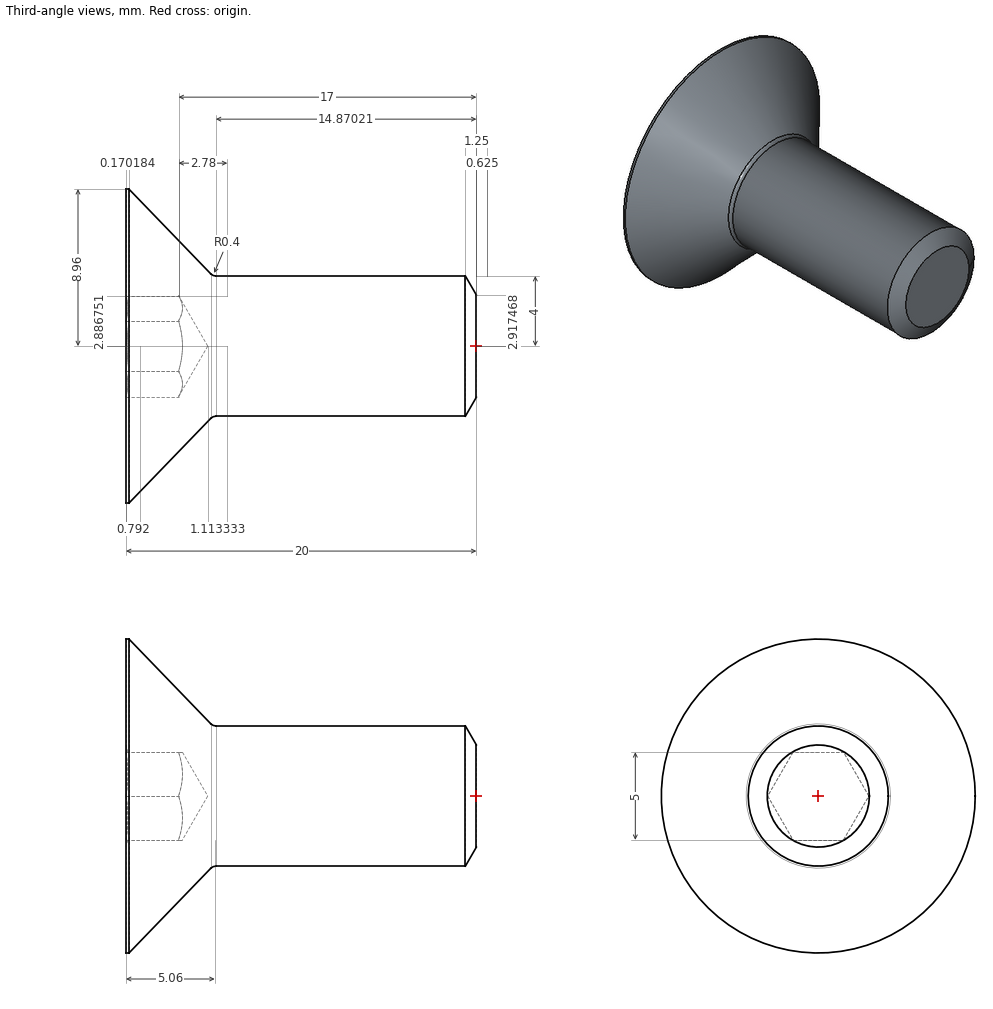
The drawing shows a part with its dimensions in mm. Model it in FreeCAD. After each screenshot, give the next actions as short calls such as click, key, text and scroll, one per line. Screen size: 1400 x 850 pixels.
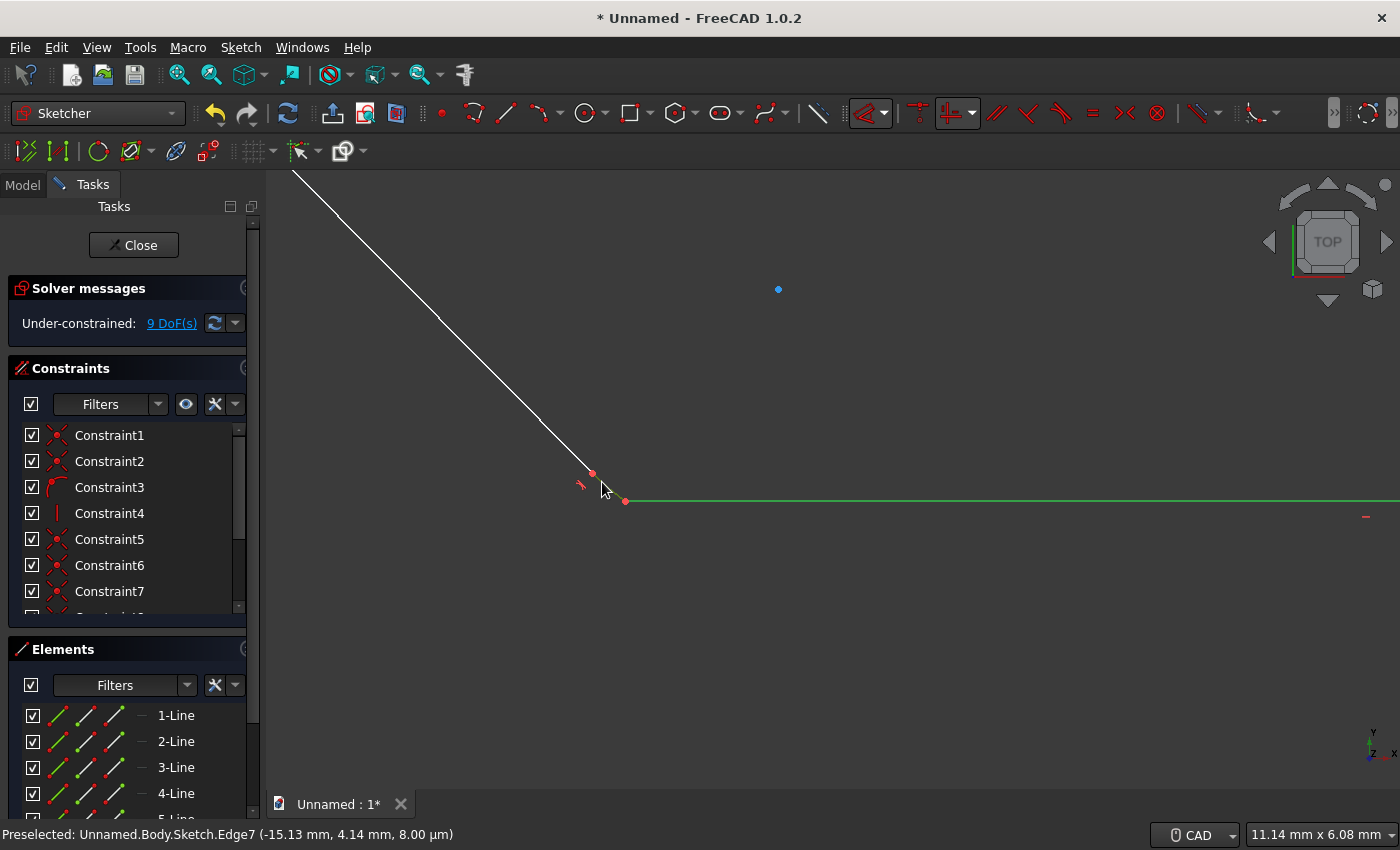
click(1062, 114)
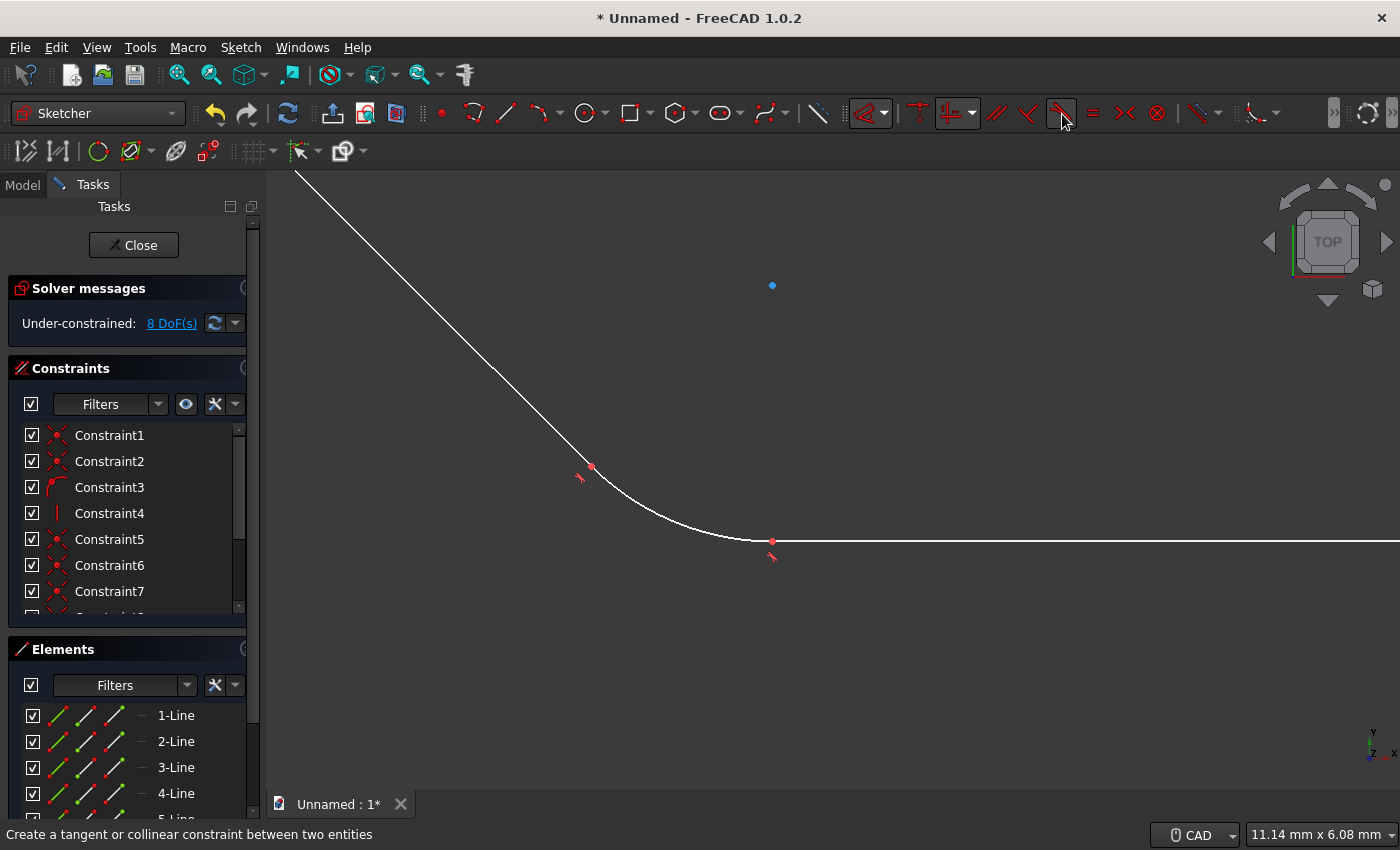
scroll(611, 494, down, 6)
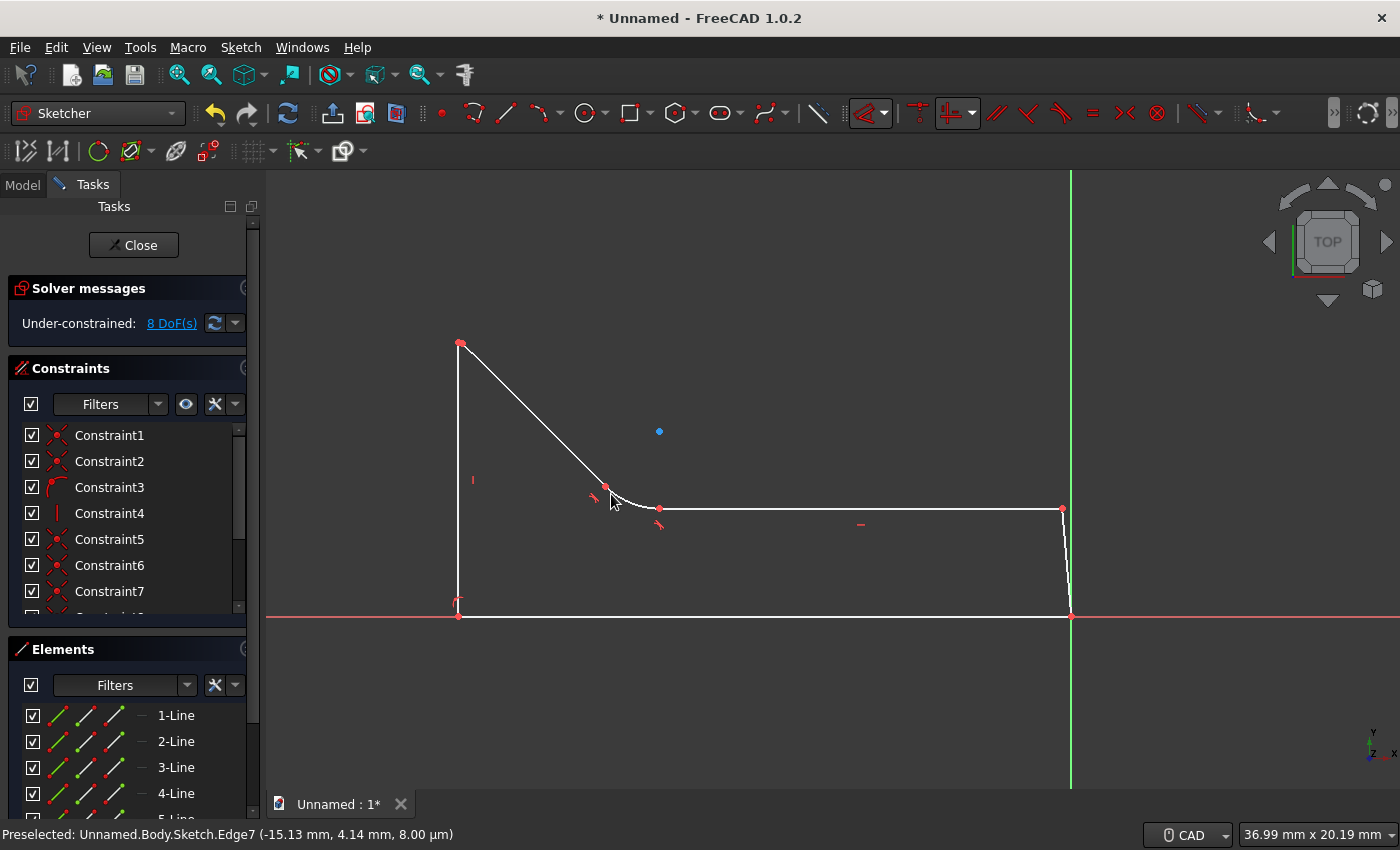
scroll(460, 343, up, 10)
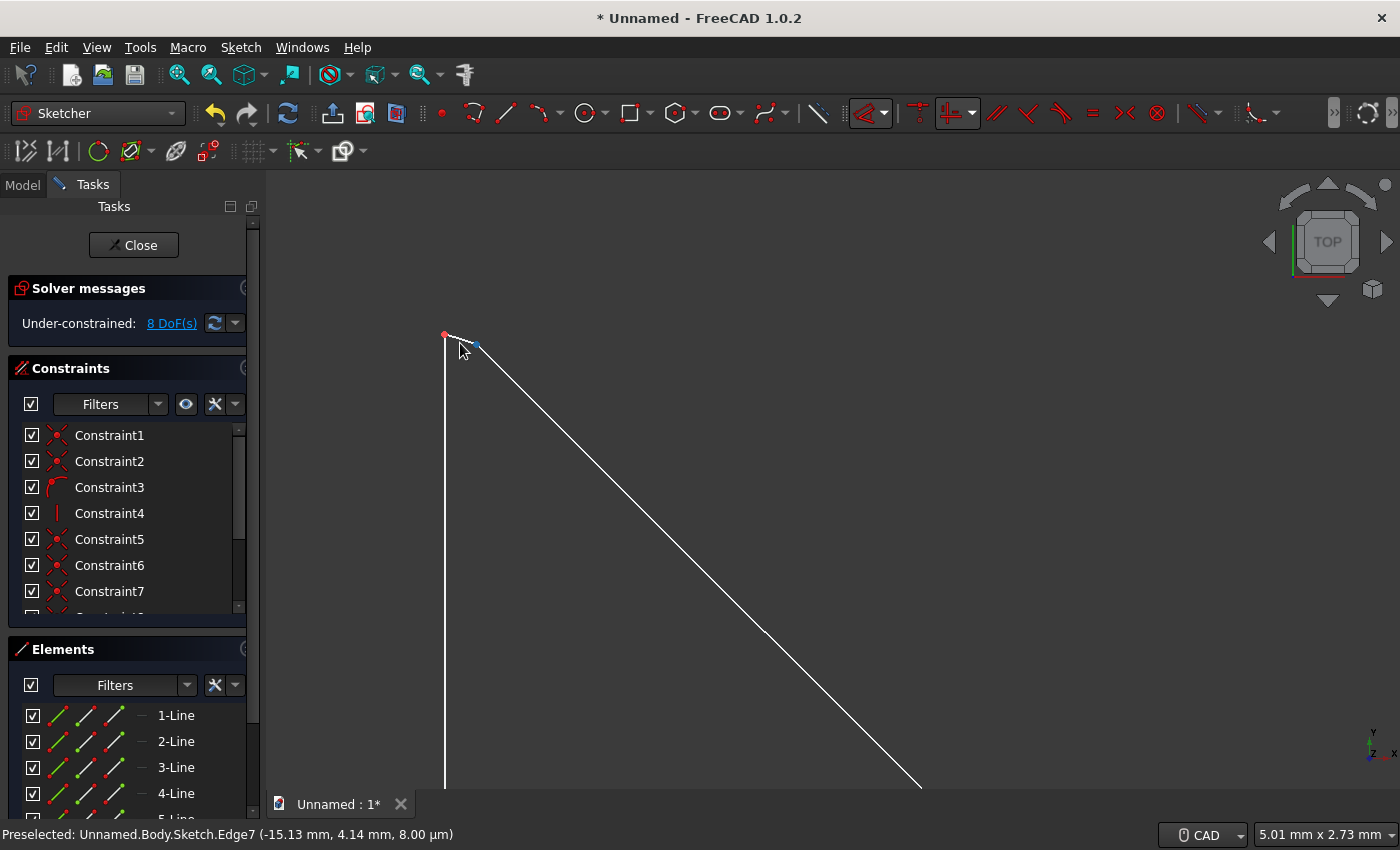
click(460, 339)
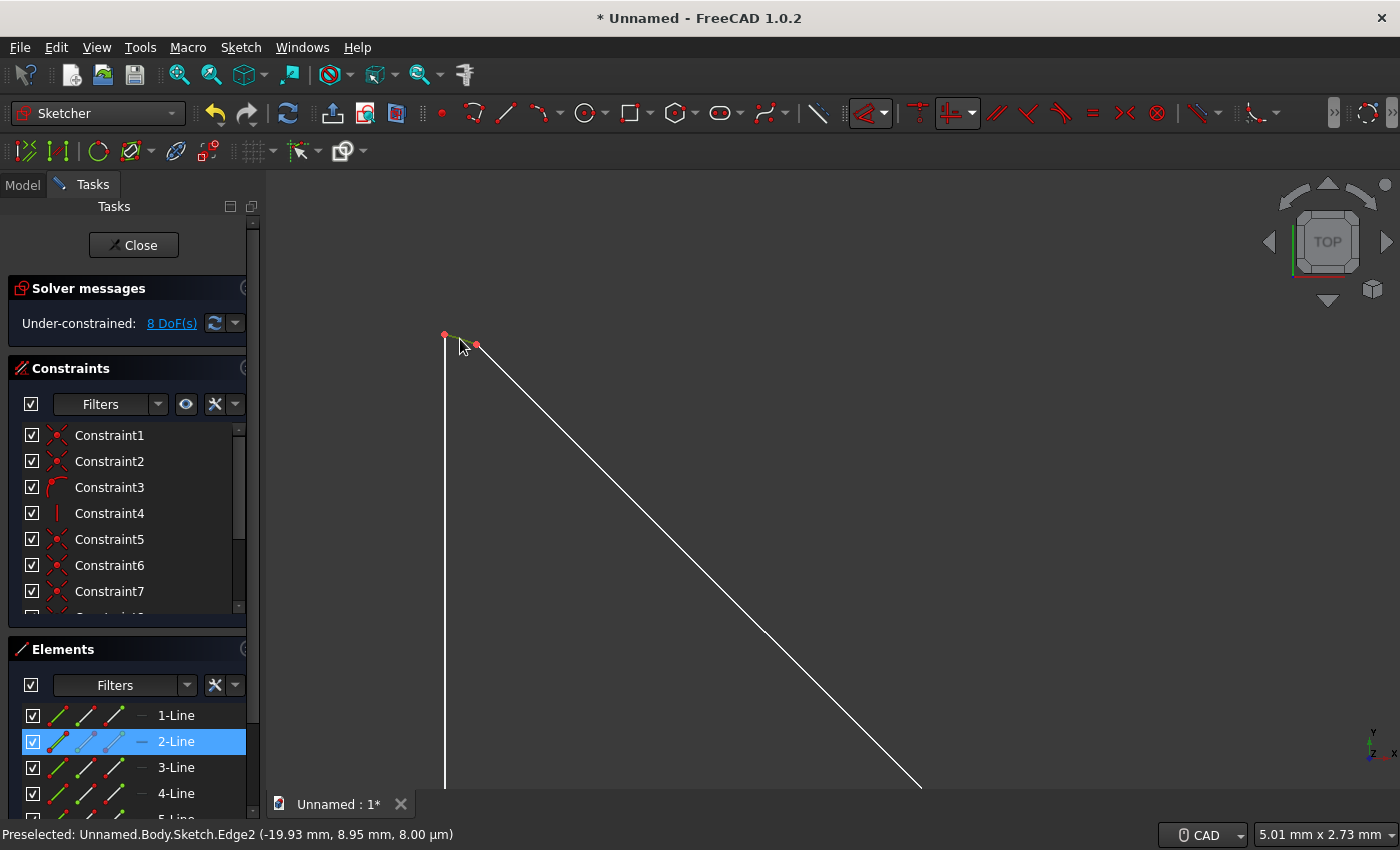
key(h)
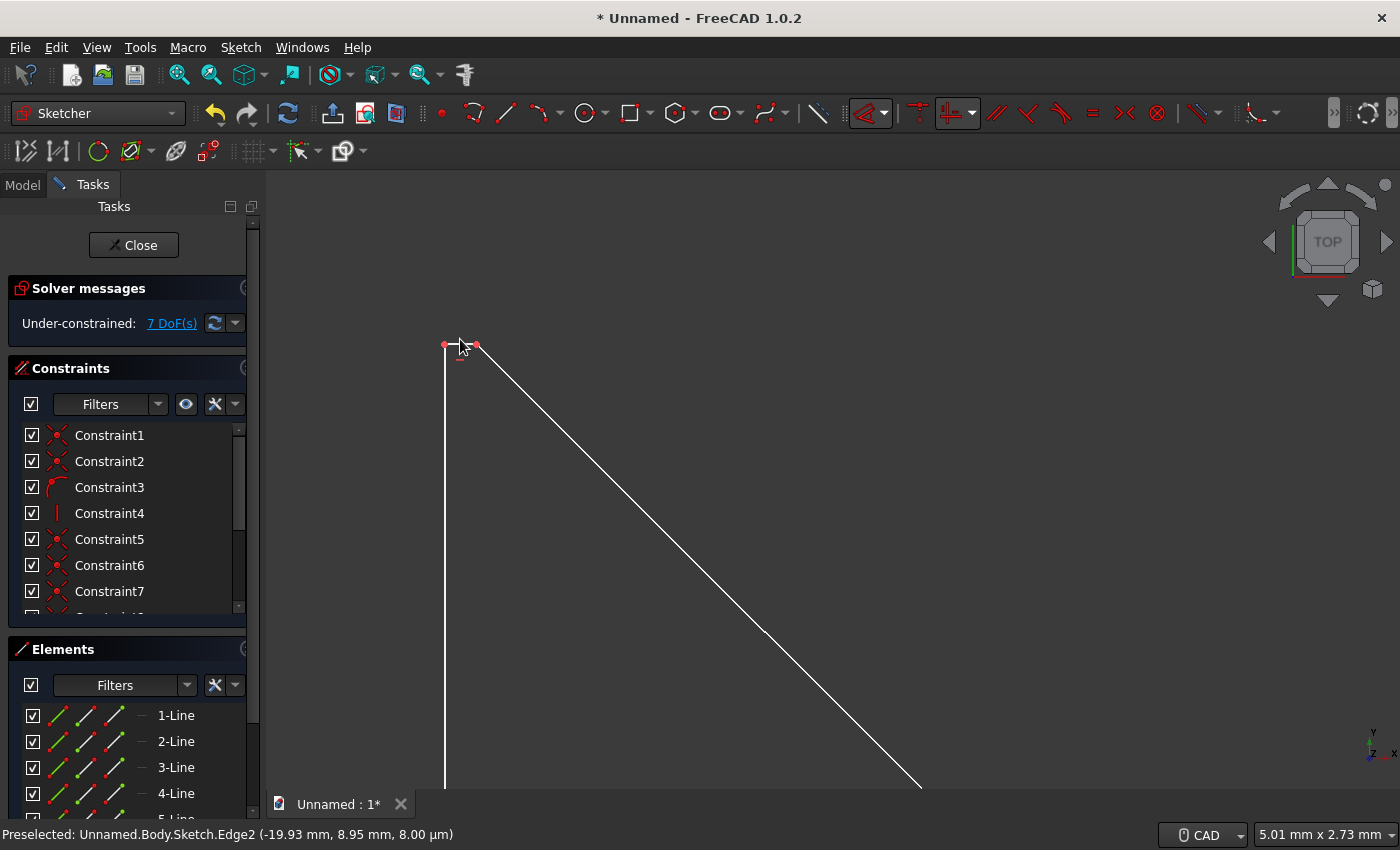
scroll(460, 343, down, 10)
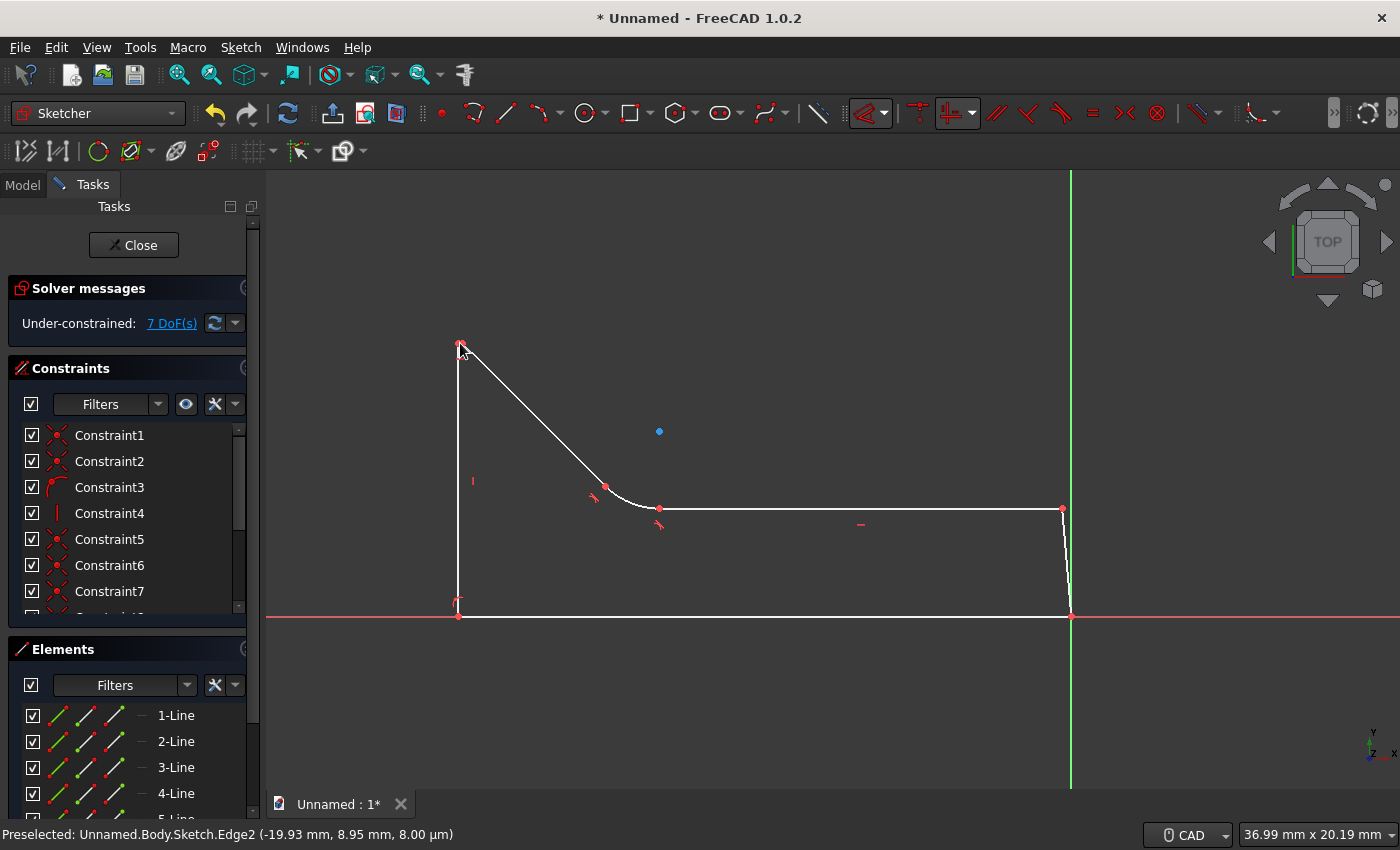
scroll(1069, 584, up, 9)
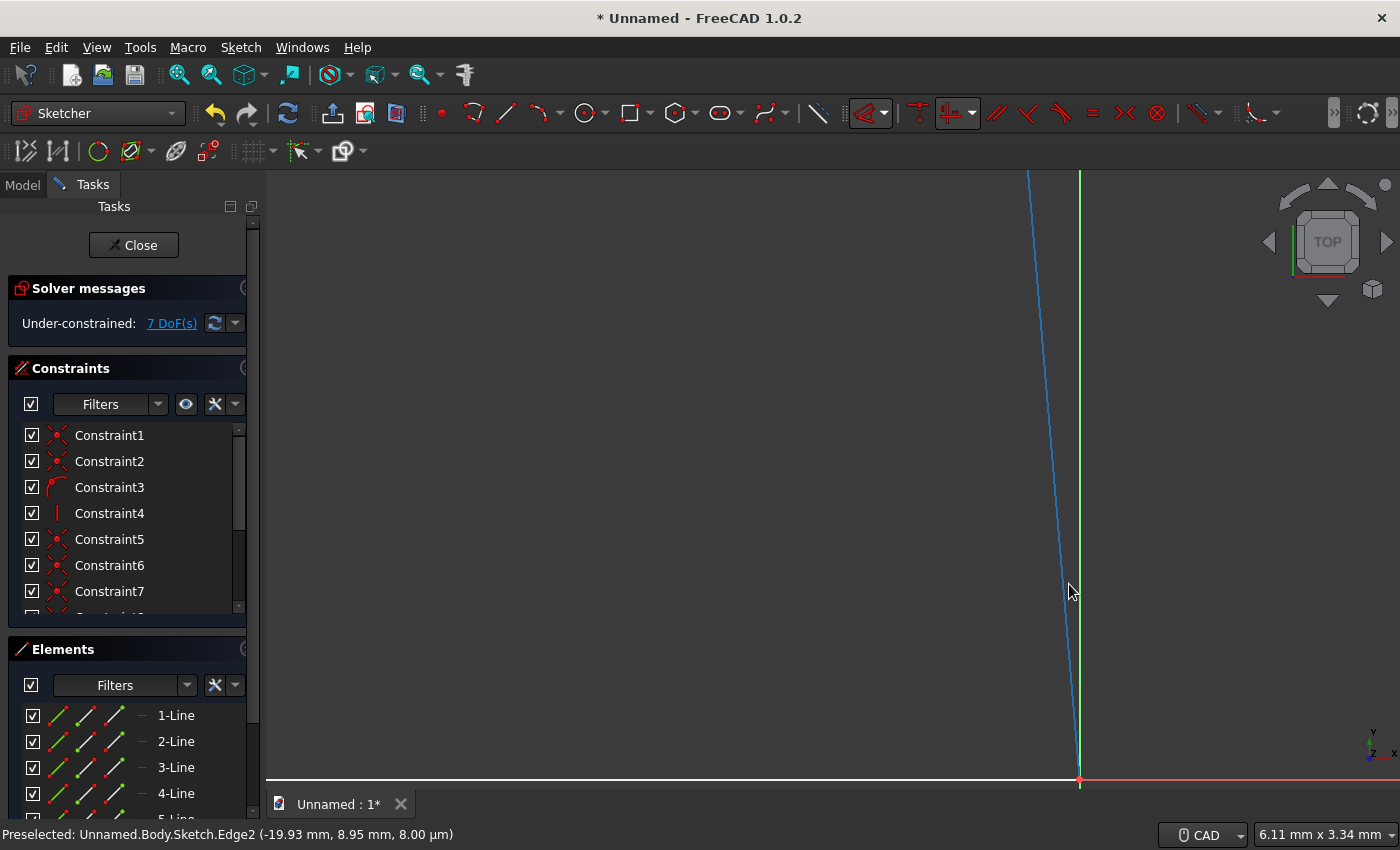
click(1063, 583)